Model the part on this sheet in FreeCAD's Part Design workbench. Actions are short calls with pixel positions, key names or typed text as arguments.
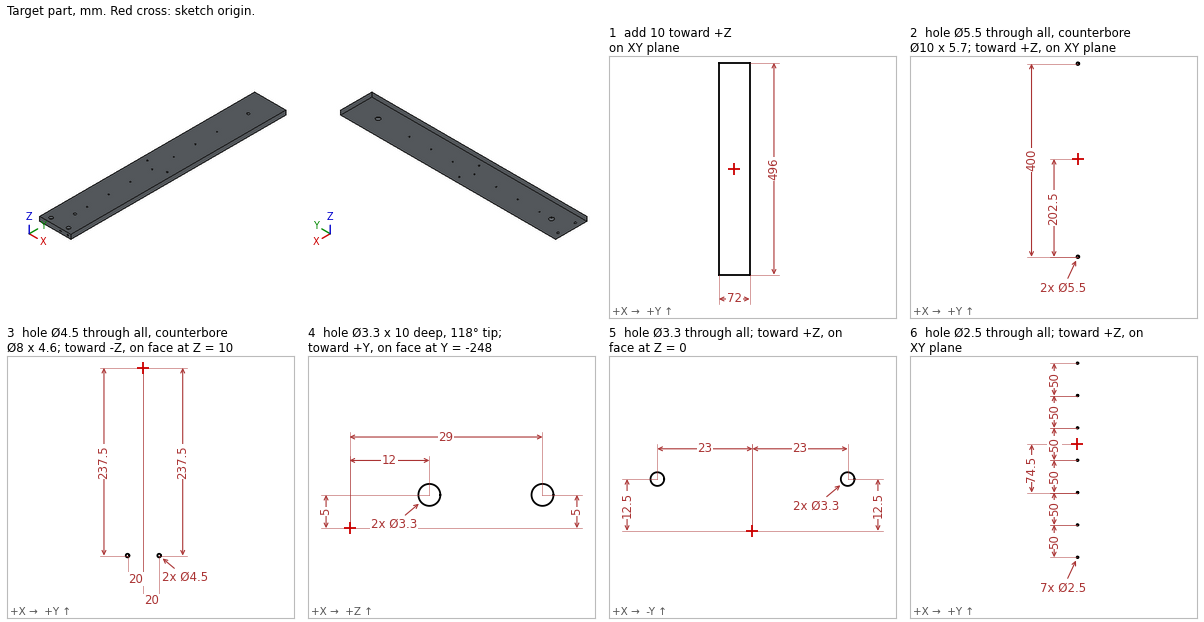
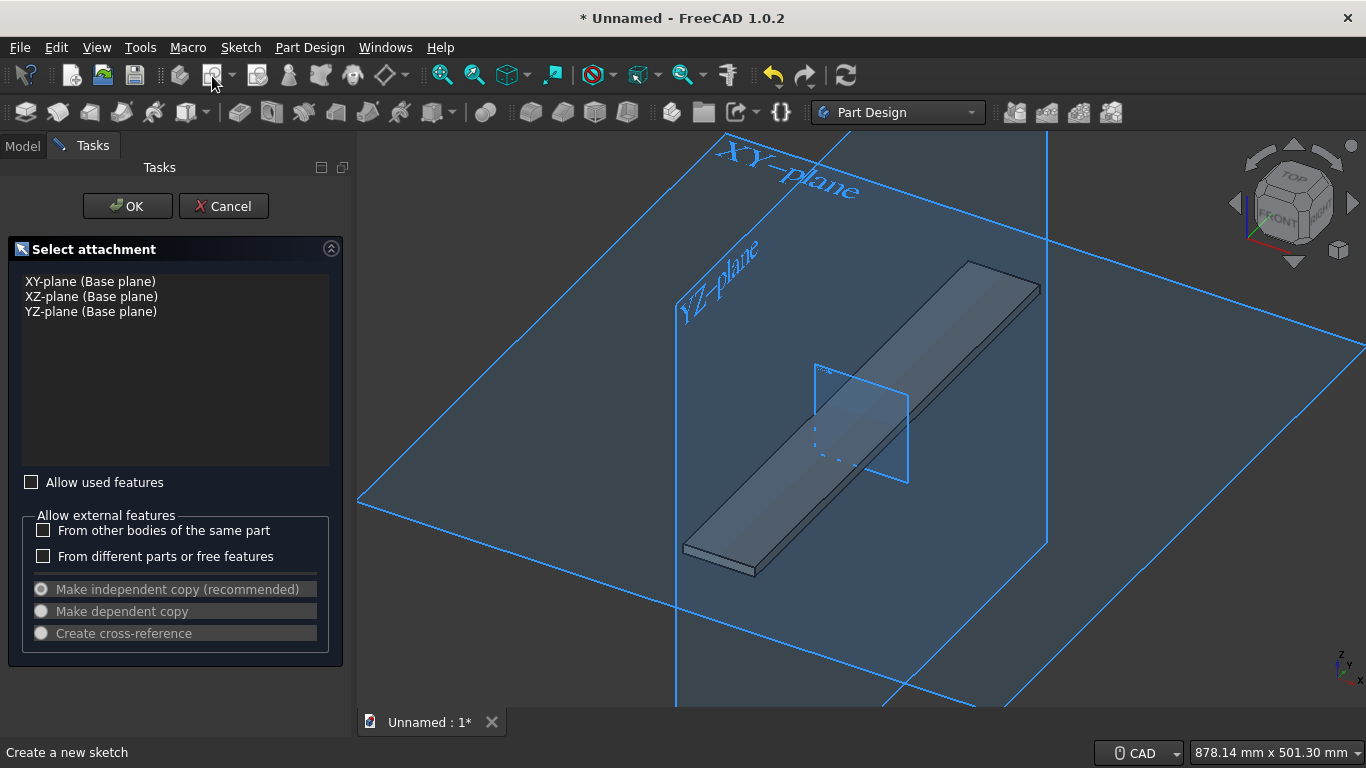
click(82, 282)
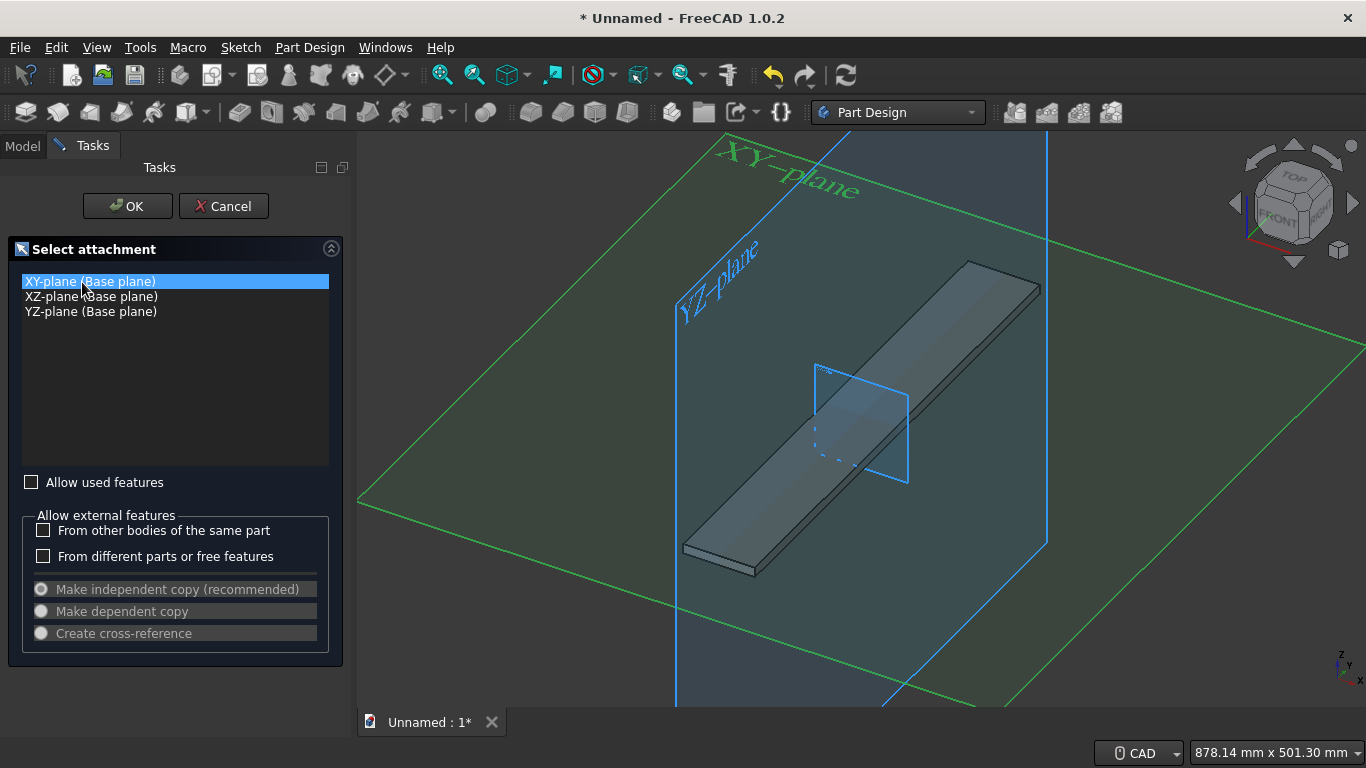
click(128, 206)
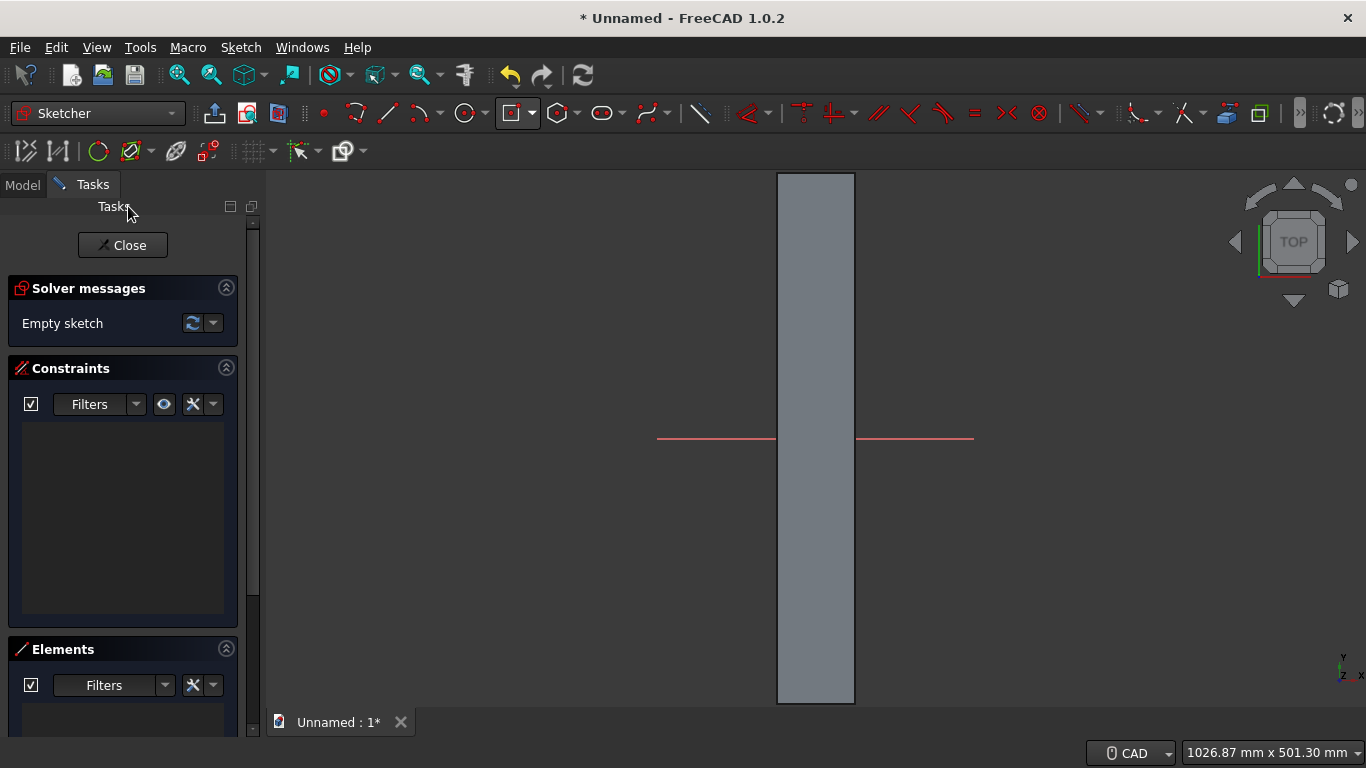
click(280, 114)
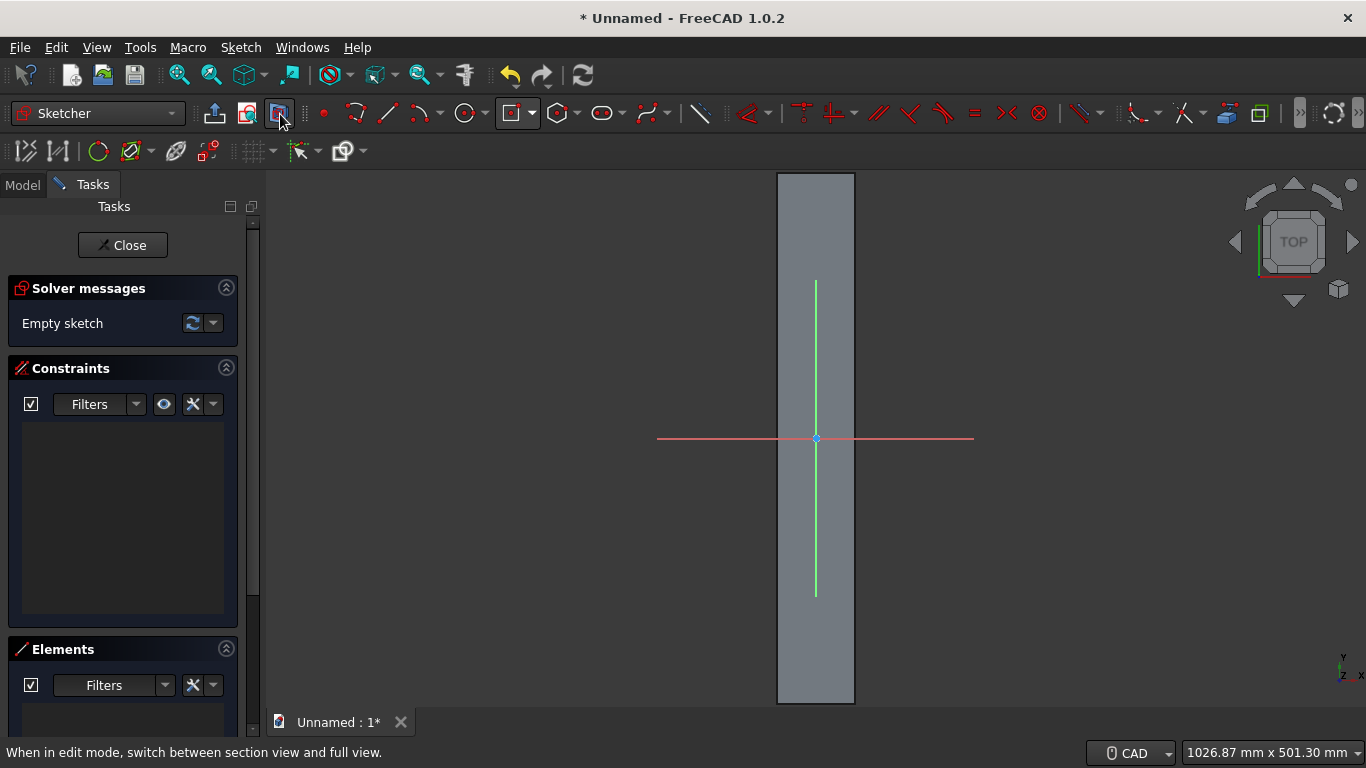
scroll(438, 426, down, 1)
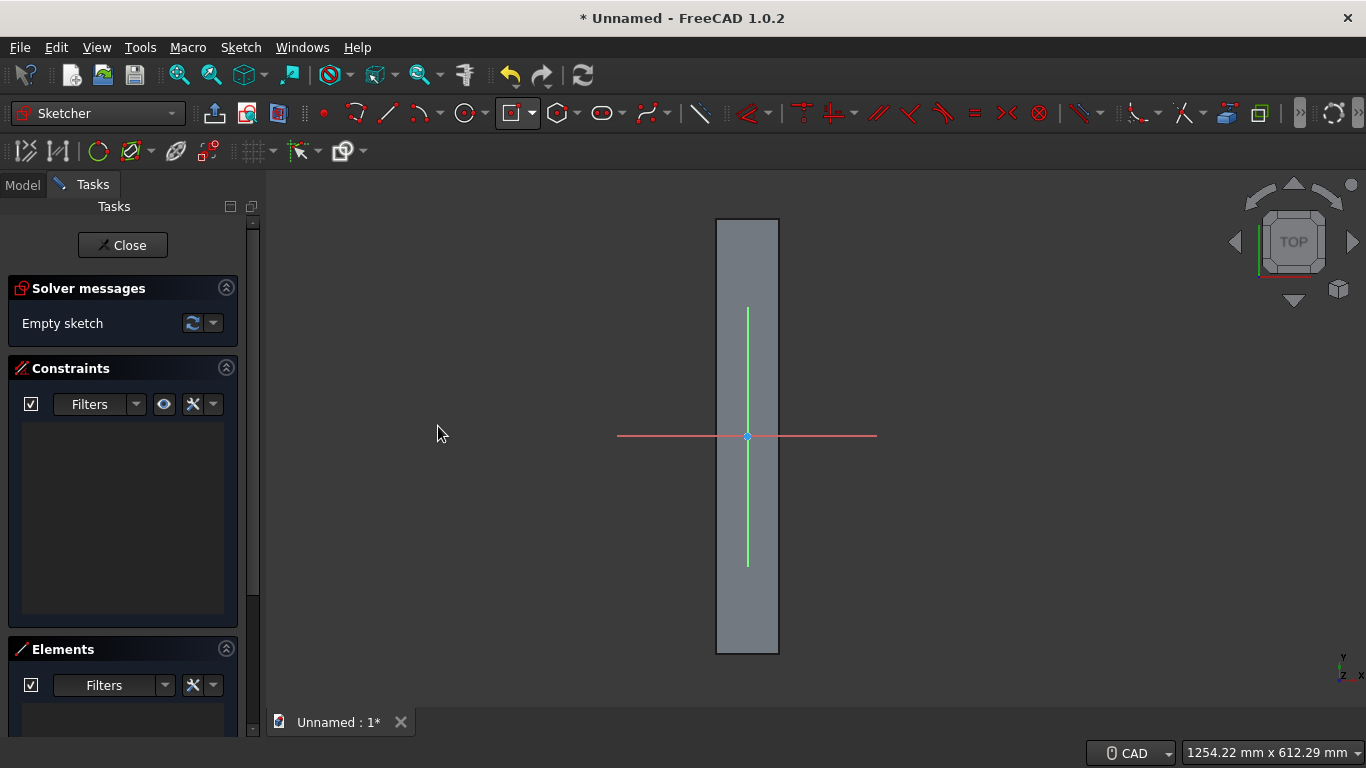
click(466, 114)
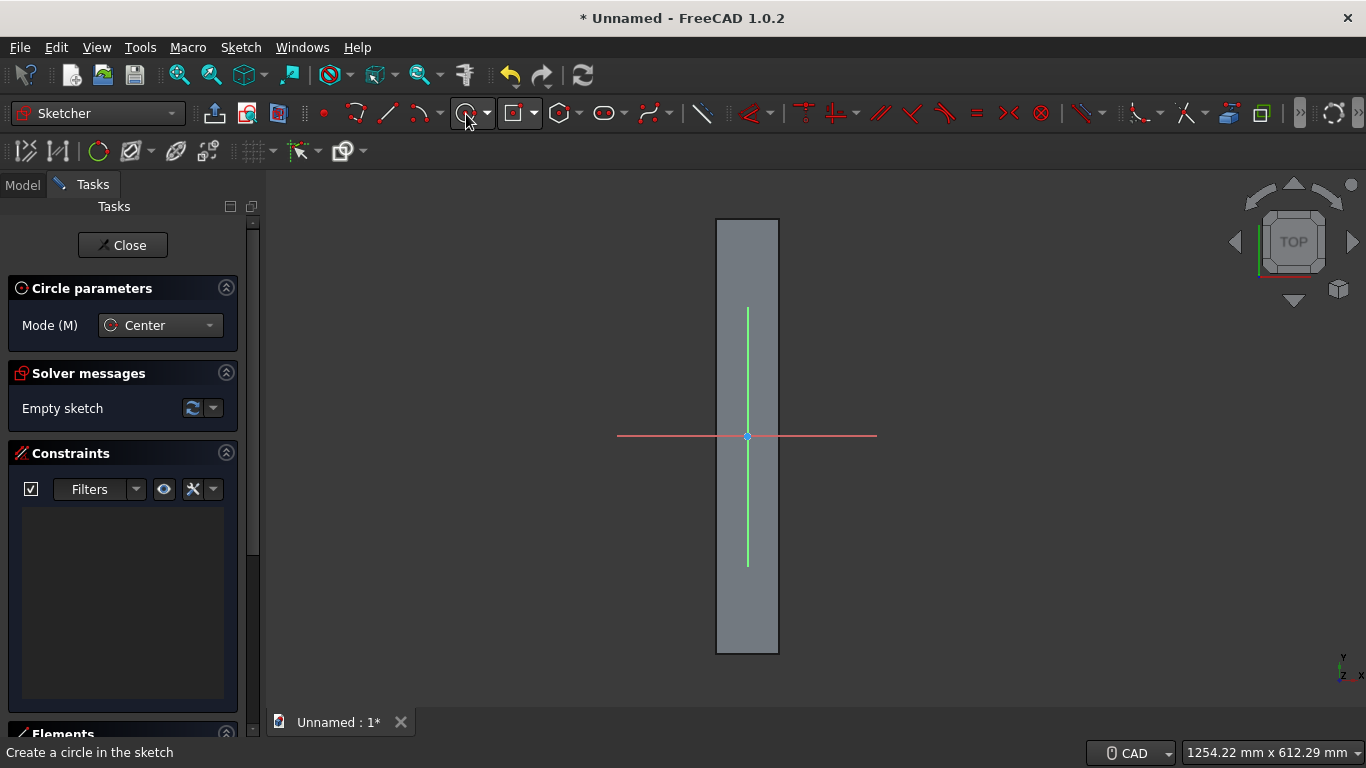
scroll(748, 614, up, 12)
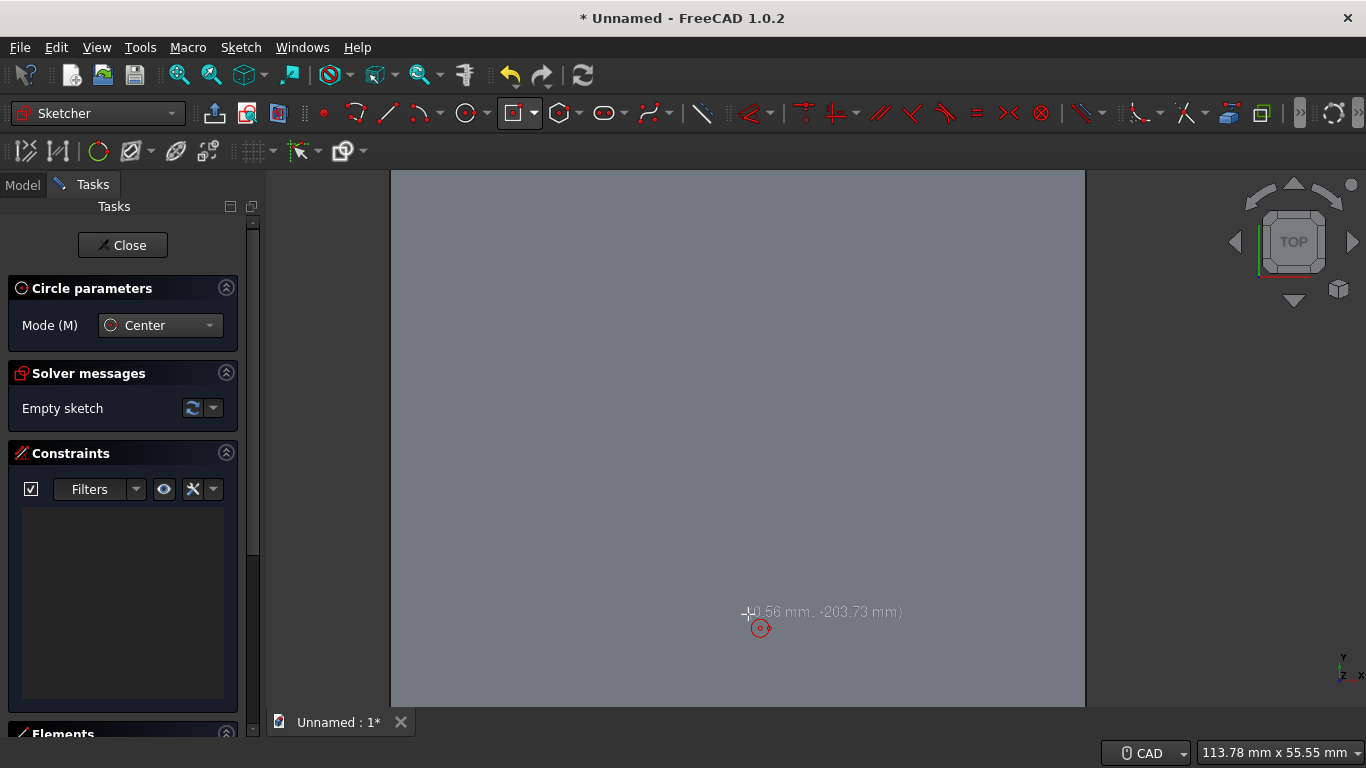
scroll(748, 615, down, 12)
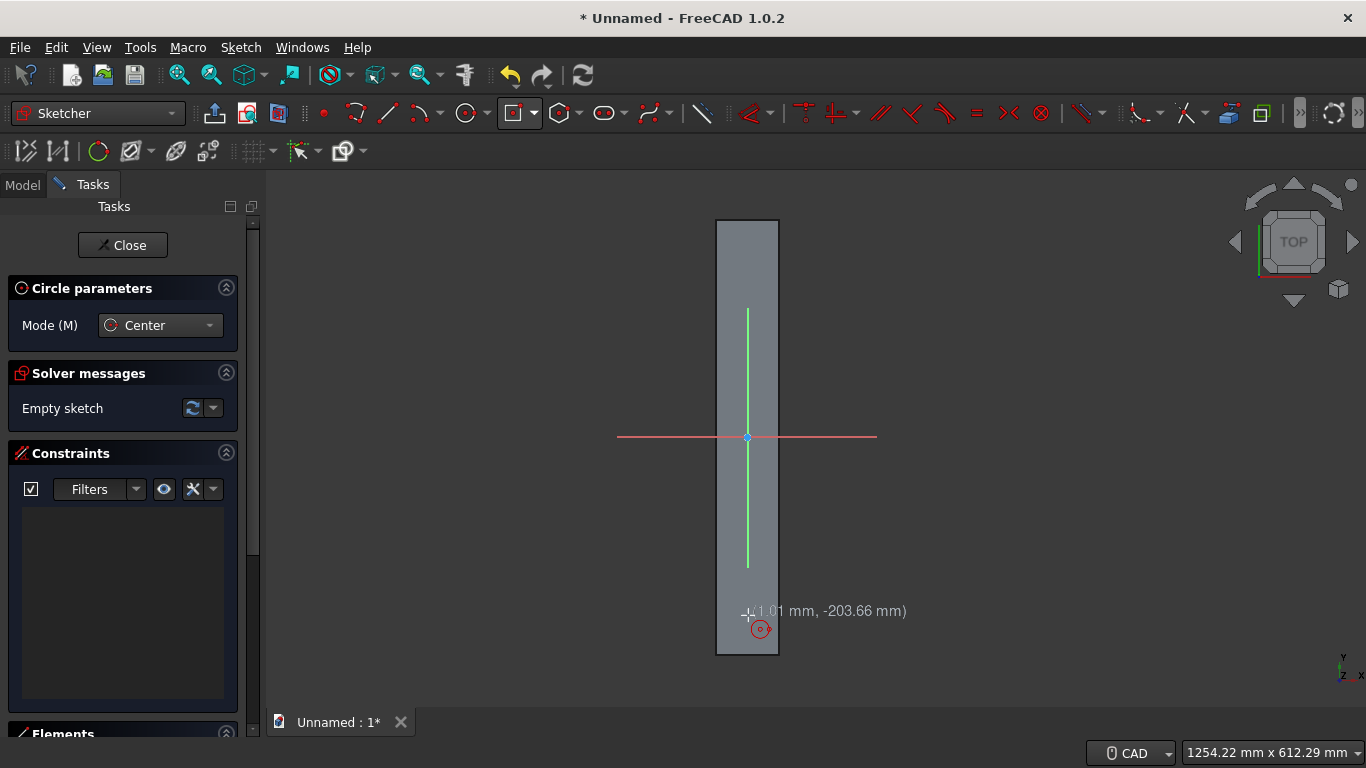
click(748, 615)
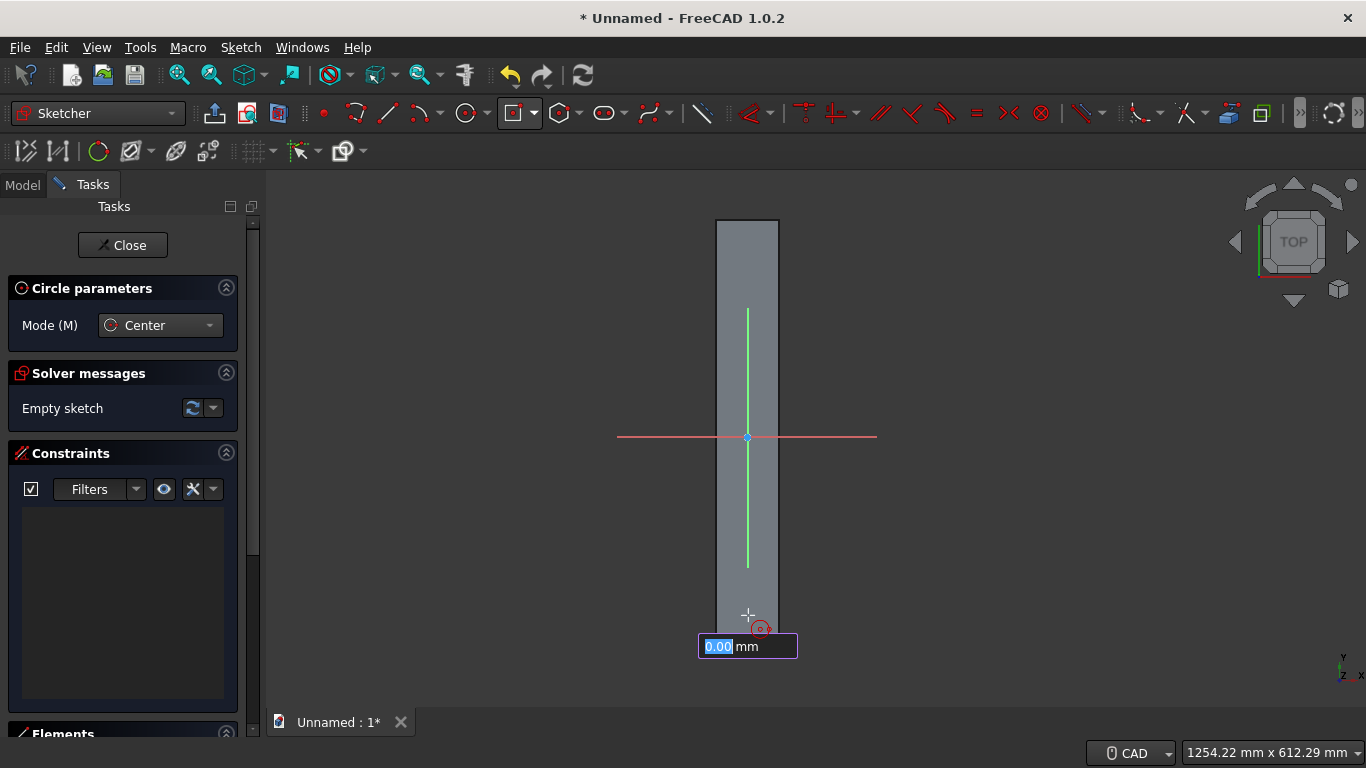
scroll(750, 614, up, 10)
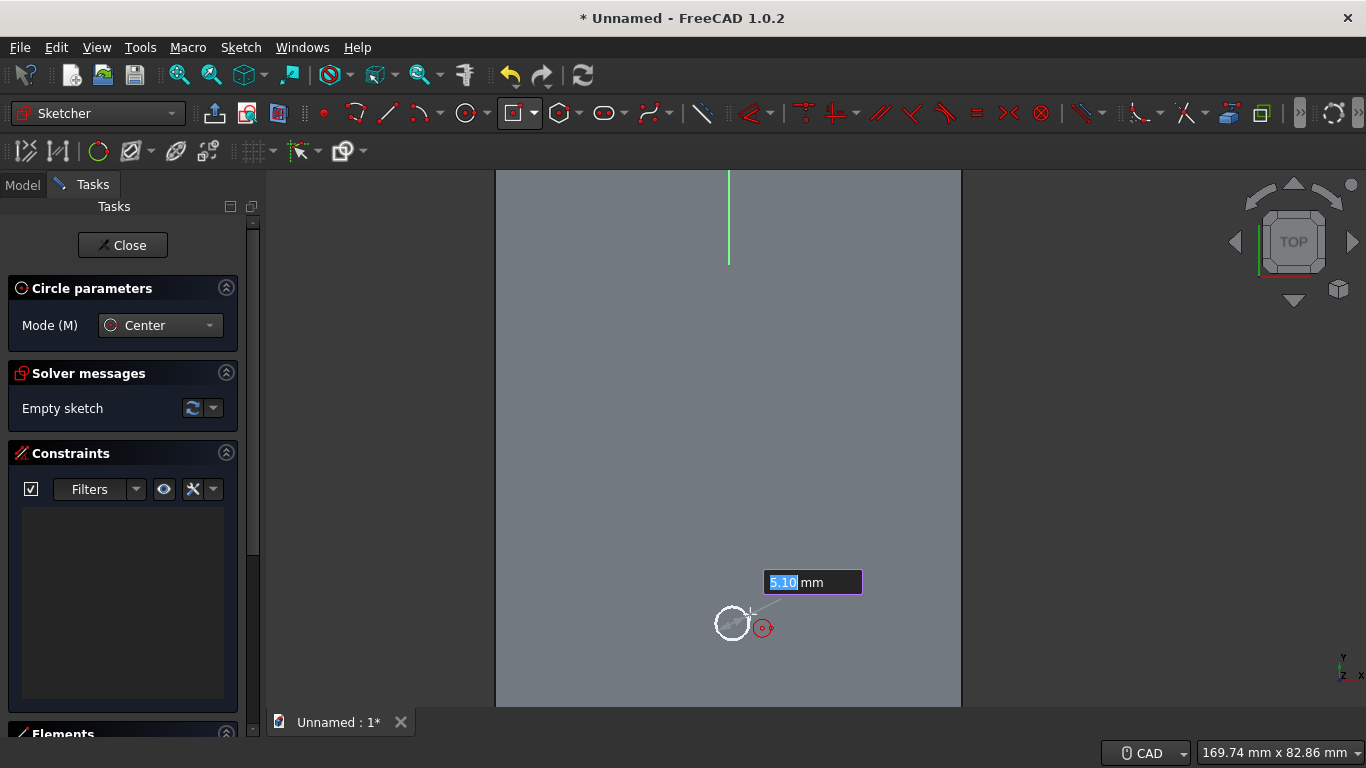
click(746, 609)